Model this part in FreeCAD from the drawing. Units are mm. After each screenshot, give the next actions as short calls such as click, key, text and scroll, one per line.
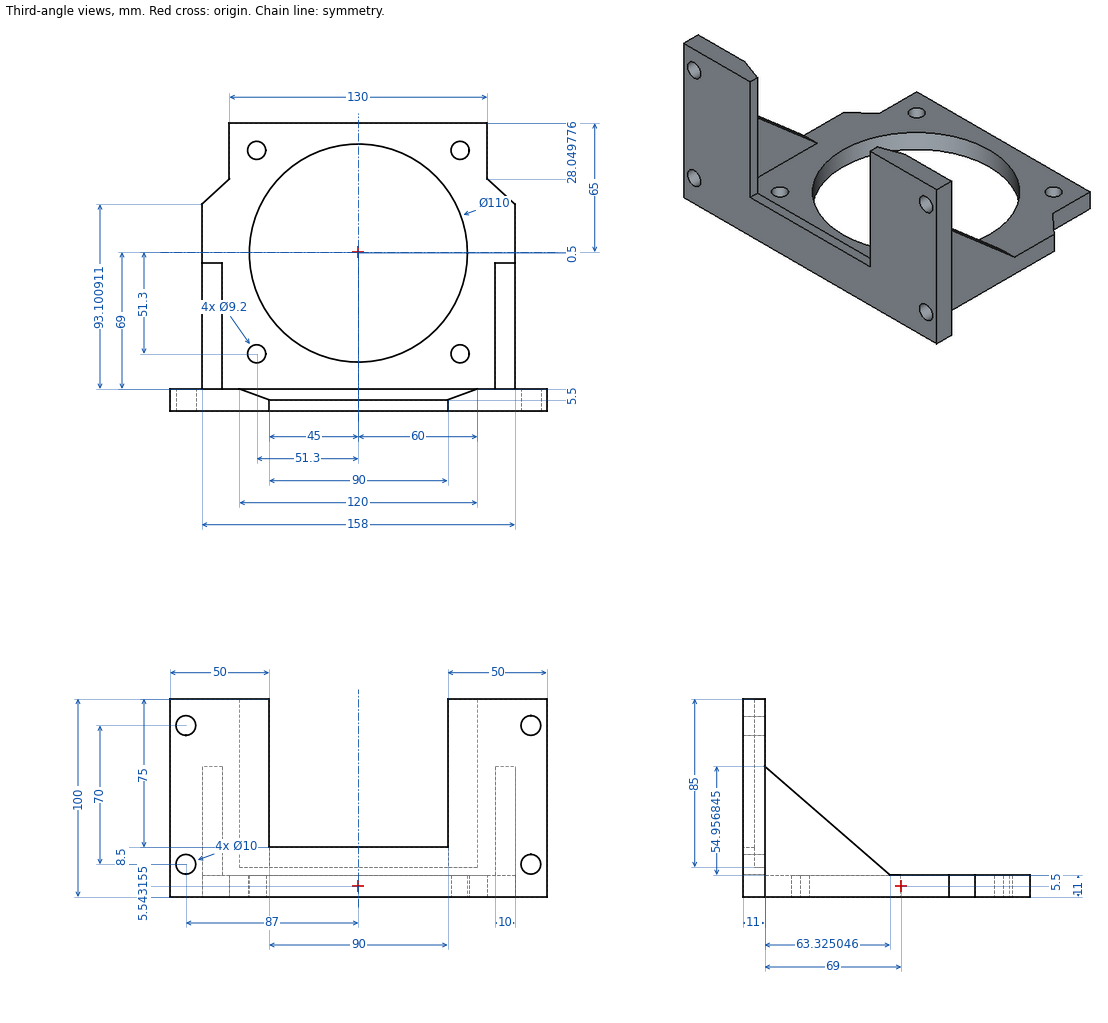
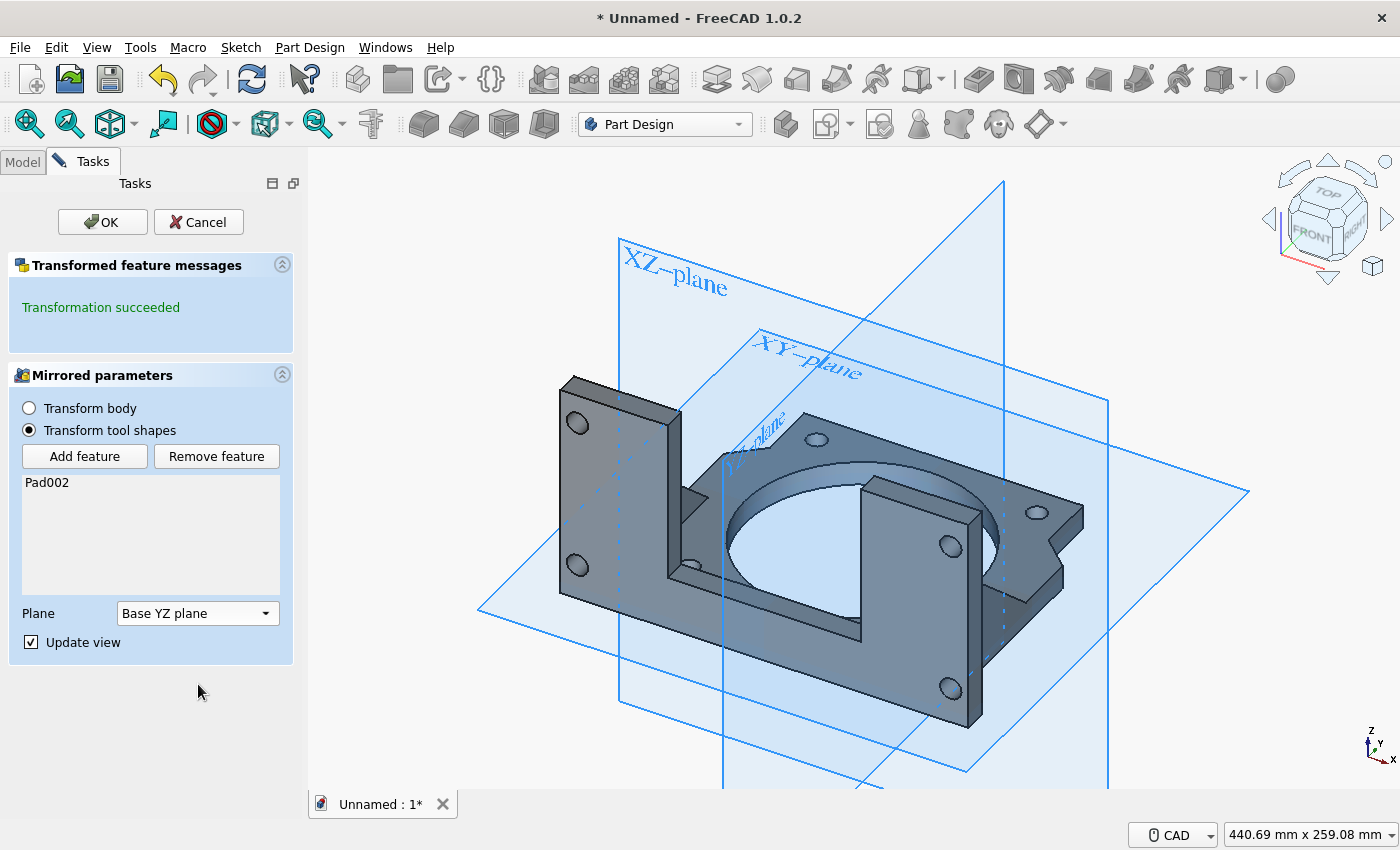
click(103, 222)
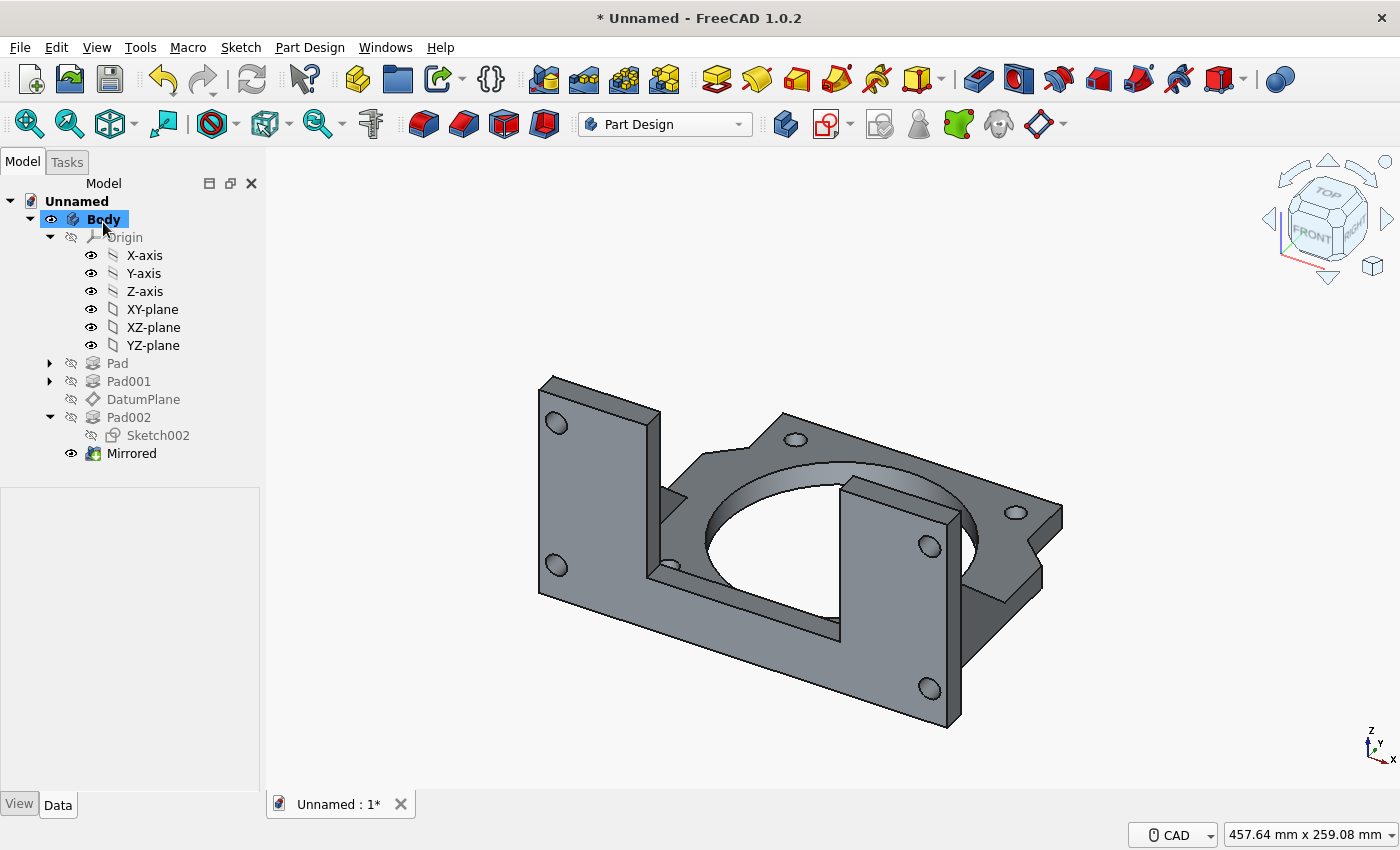
click(632, 408)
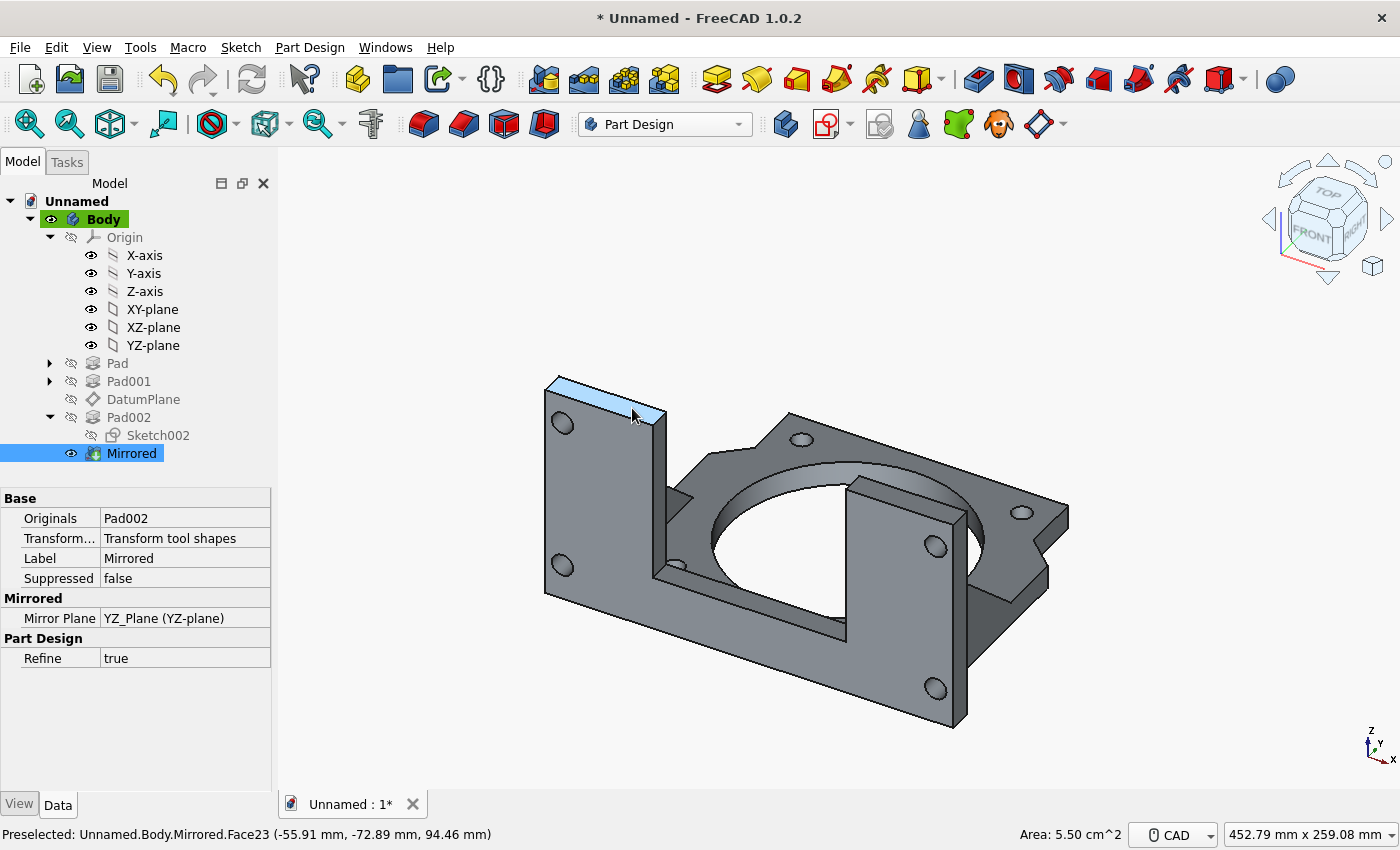
click(826, 124)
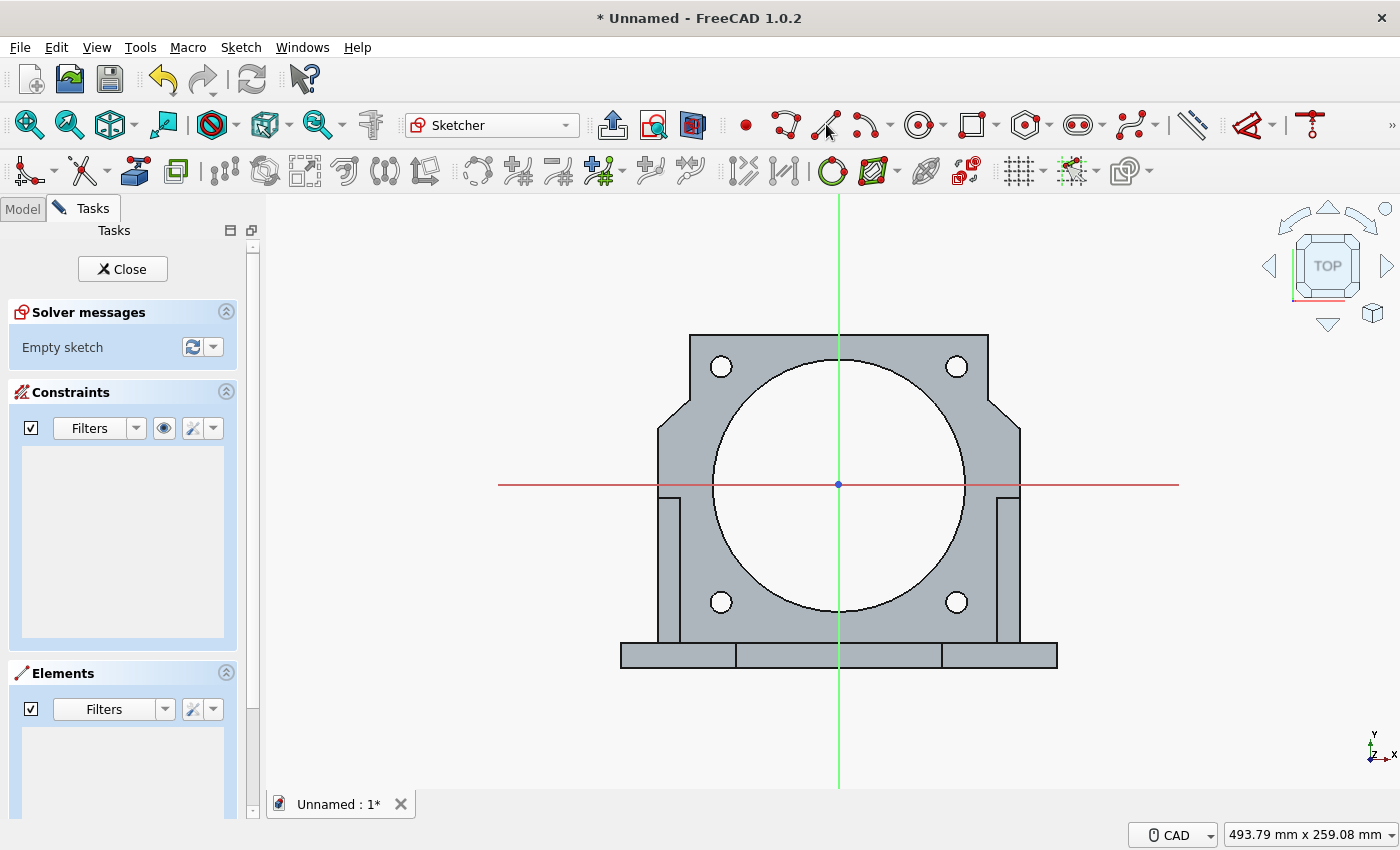
scroll(900, 634, up, 4)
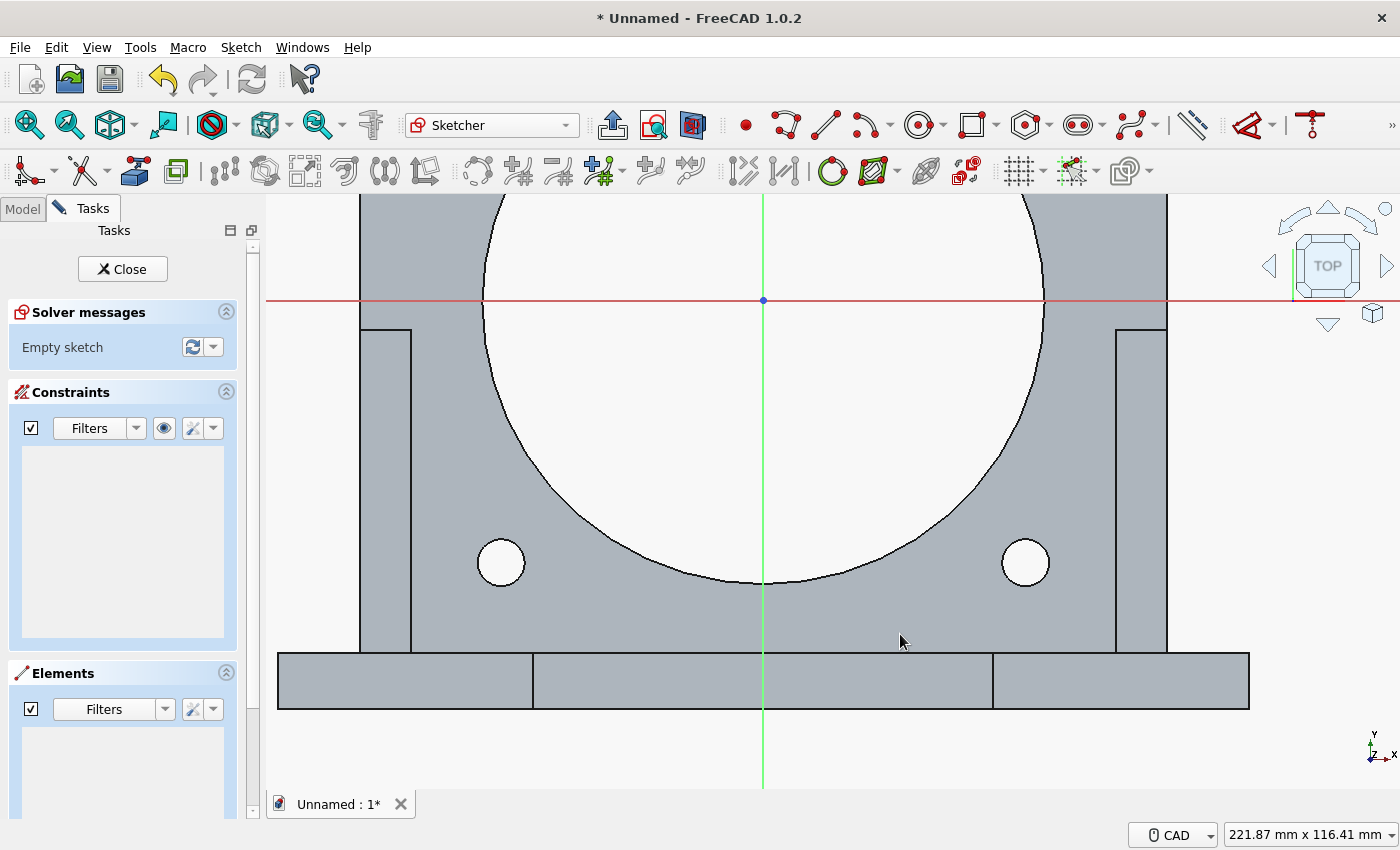
click(786, 126)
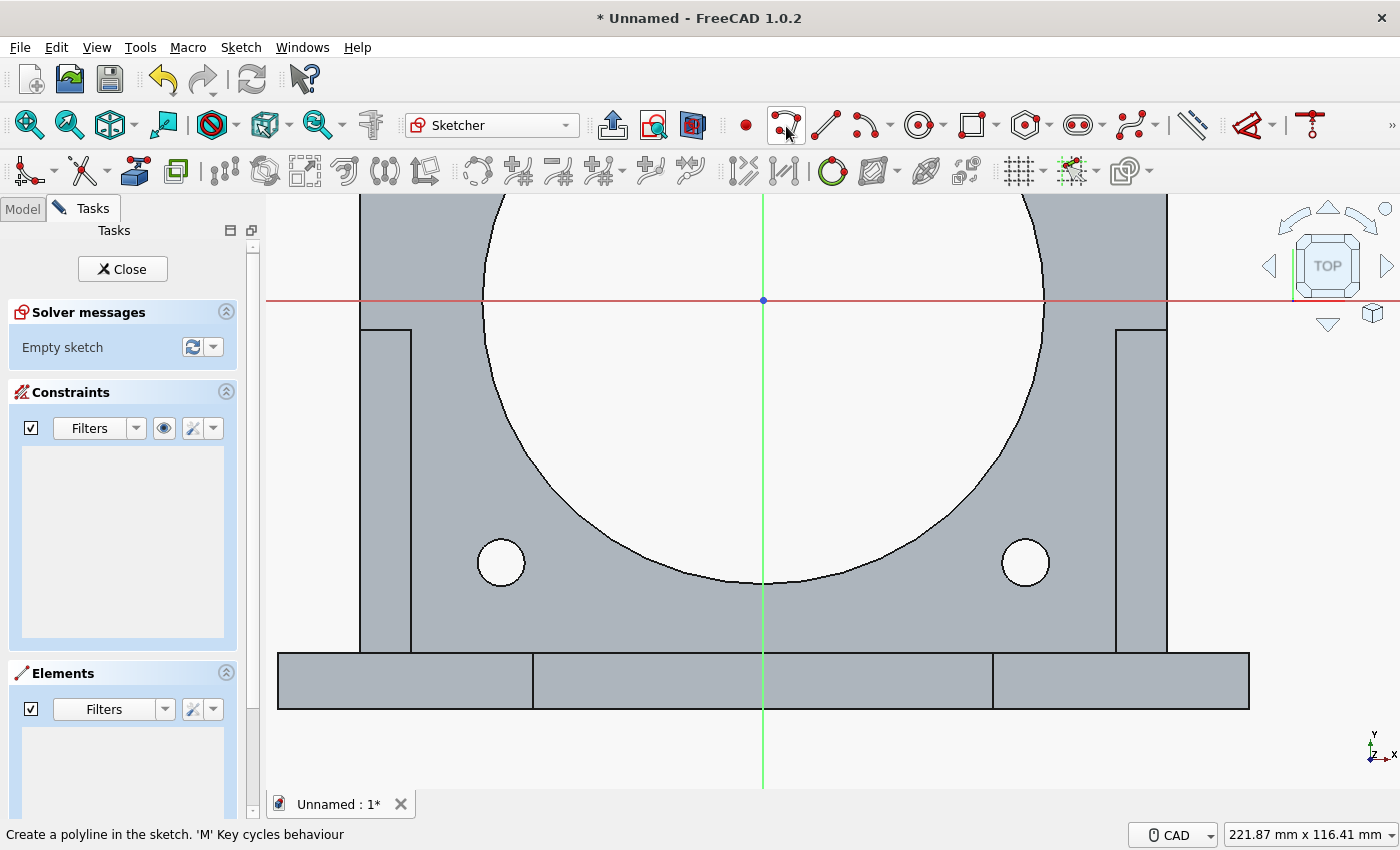
click(533, 681)
click(993, 681)
click(1070, 653)
click(457, 653)
click(533, 682)
key(Escape)
key(Escape)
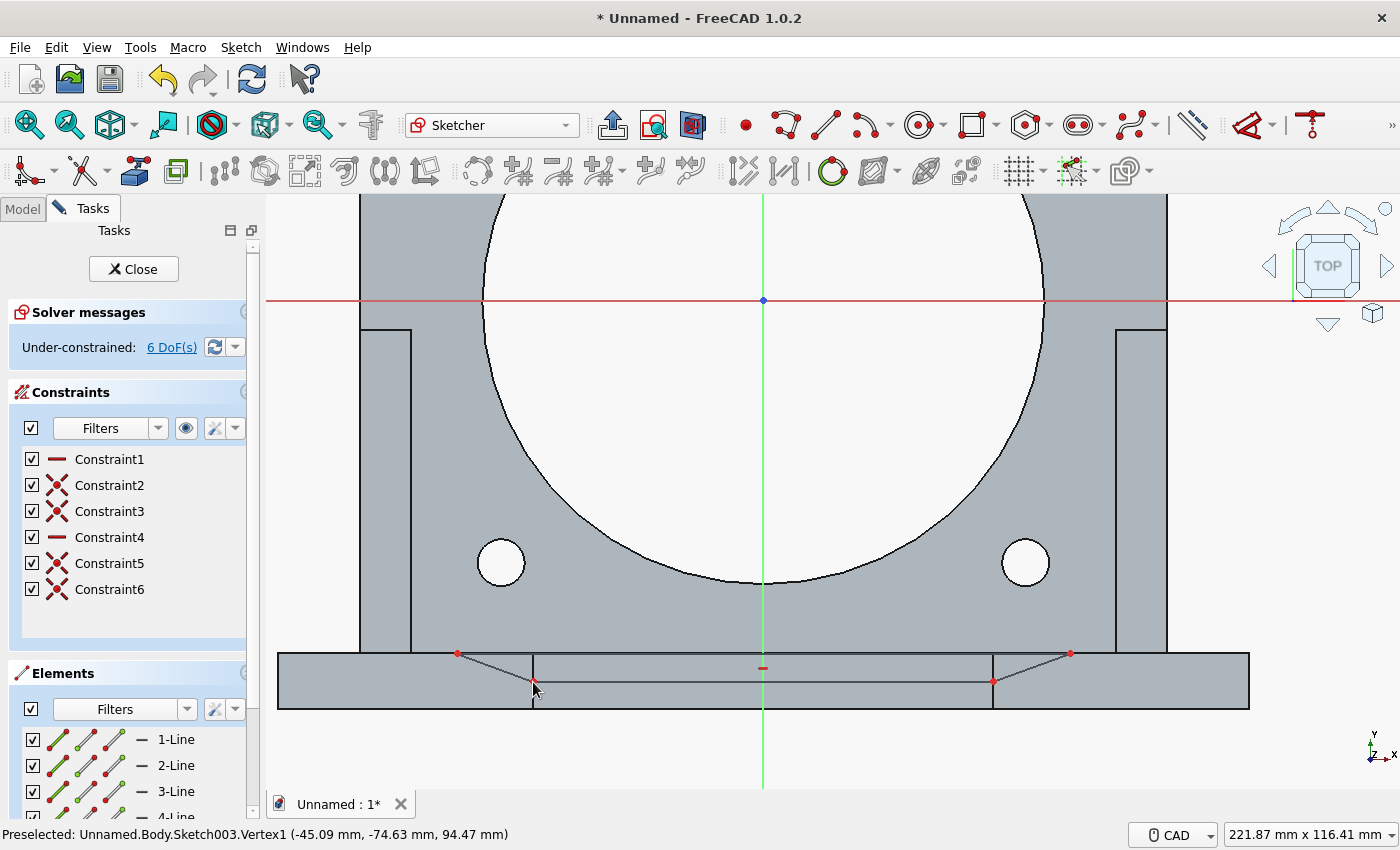
click(1248, 126)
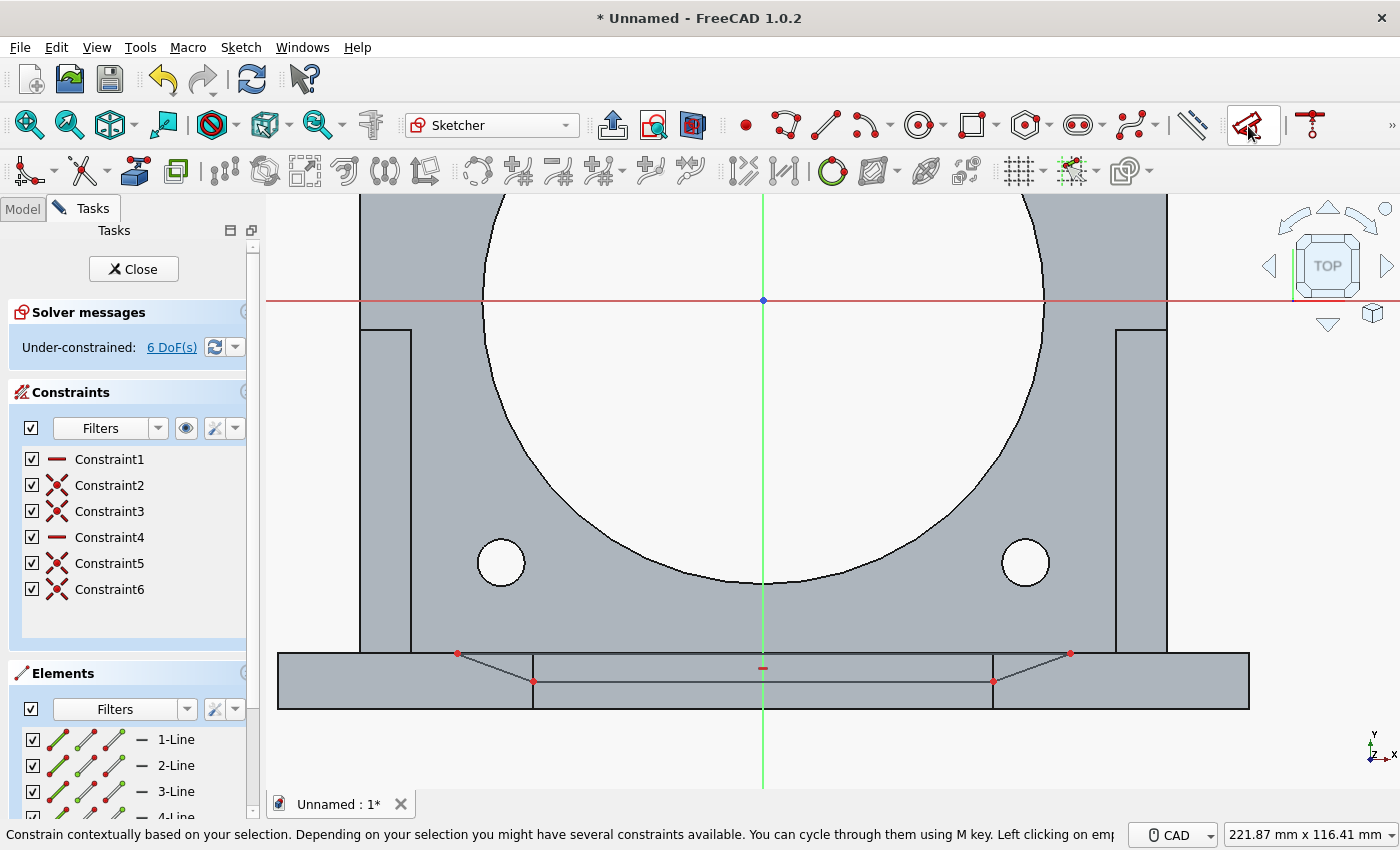
click(671, 682)
click(657, 716)